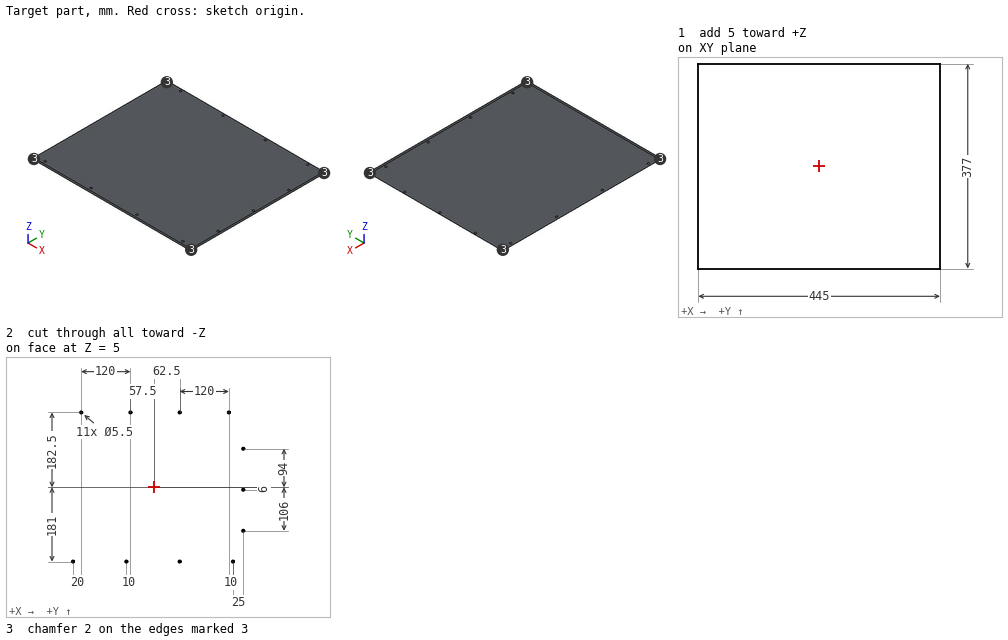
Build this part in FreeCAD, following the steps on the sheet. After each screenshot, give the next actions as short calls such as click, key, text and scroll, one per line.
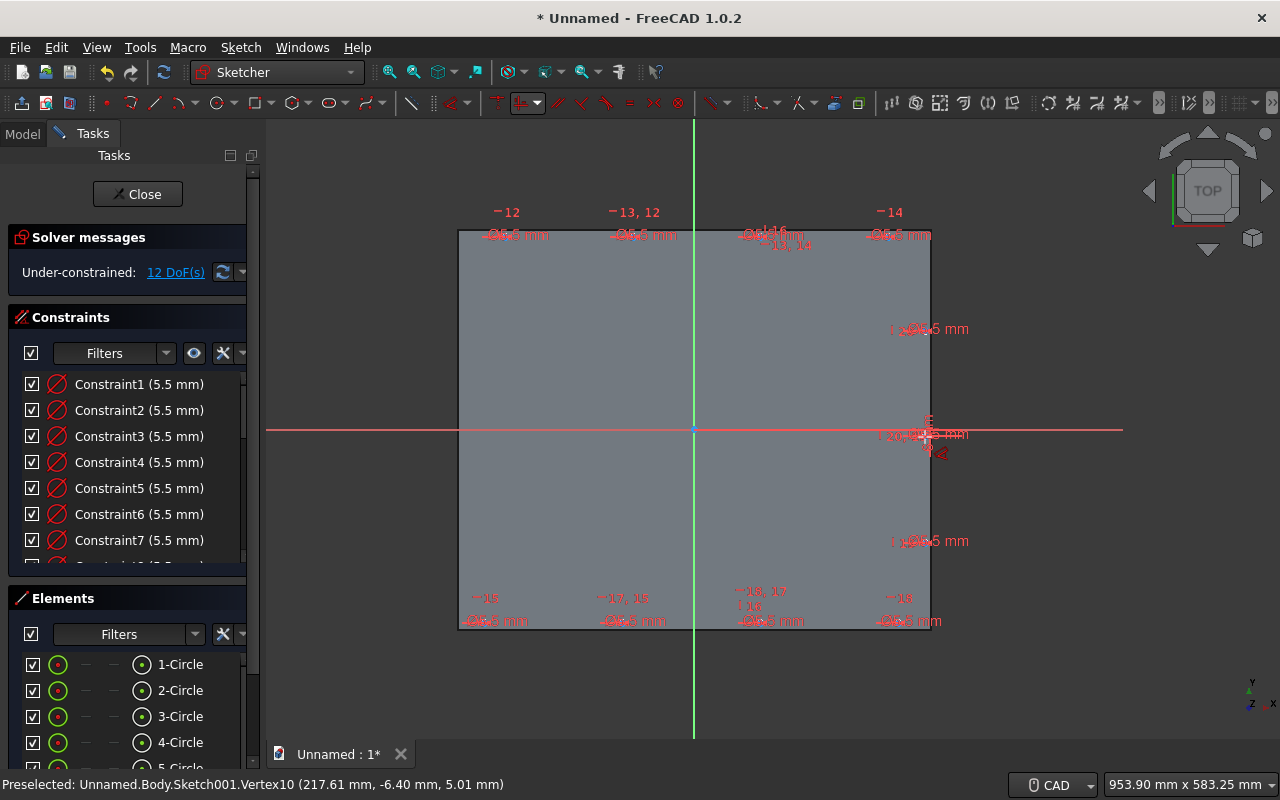
click(925, 331)
click(959, 380)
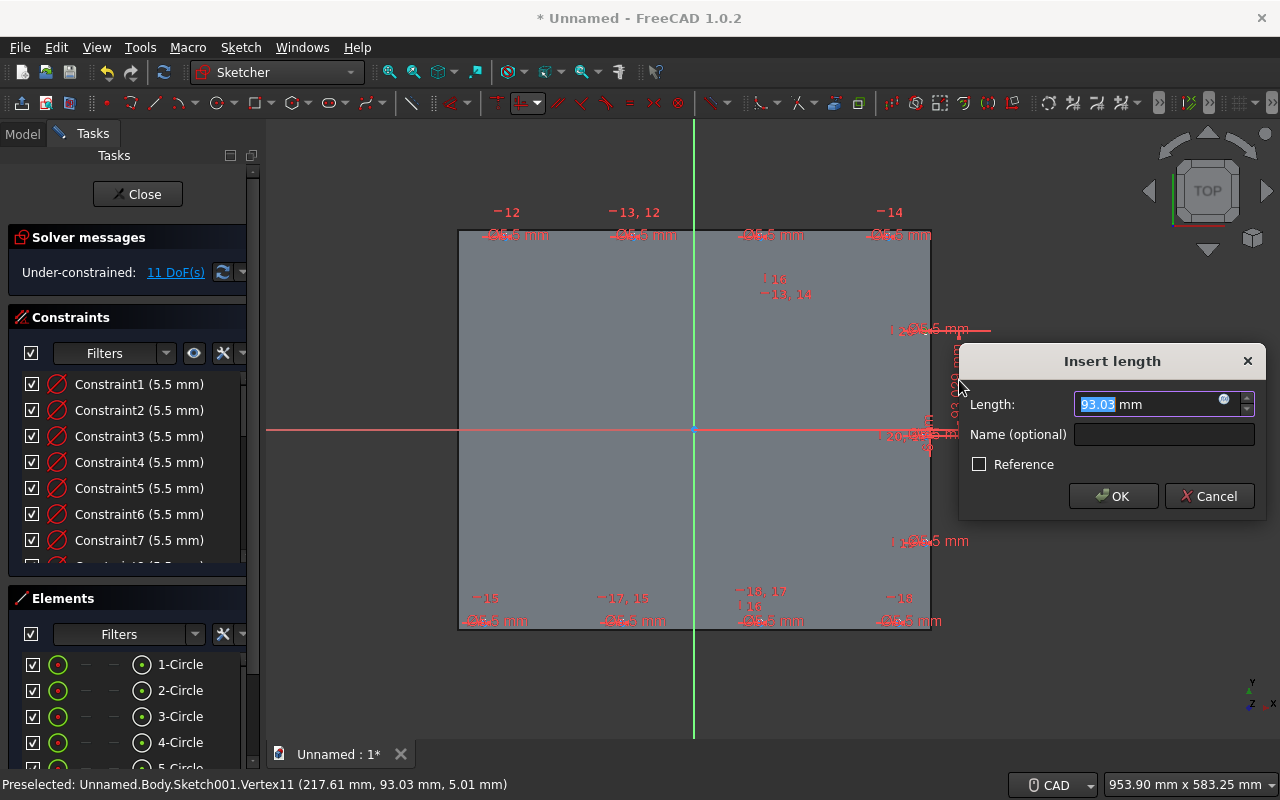
text(94)
key(Return)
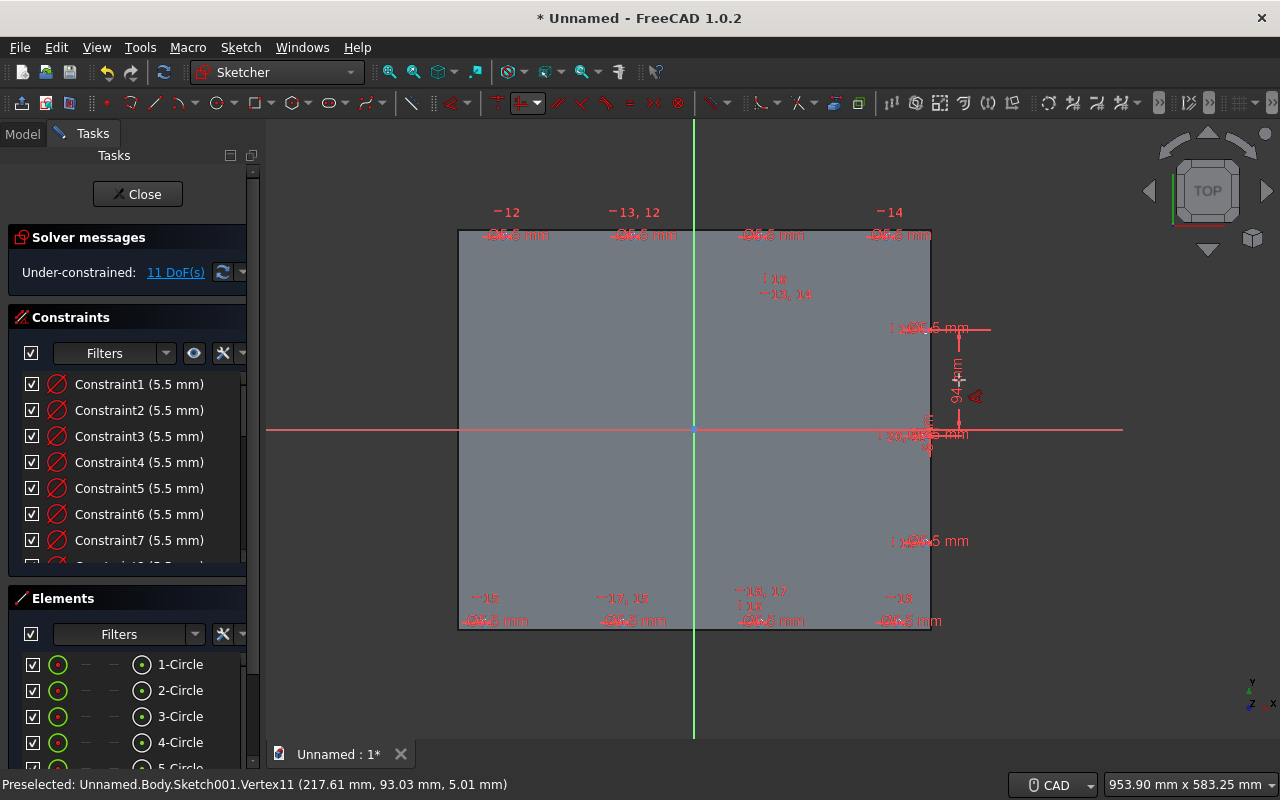
click(484, 623)
click(450, 526)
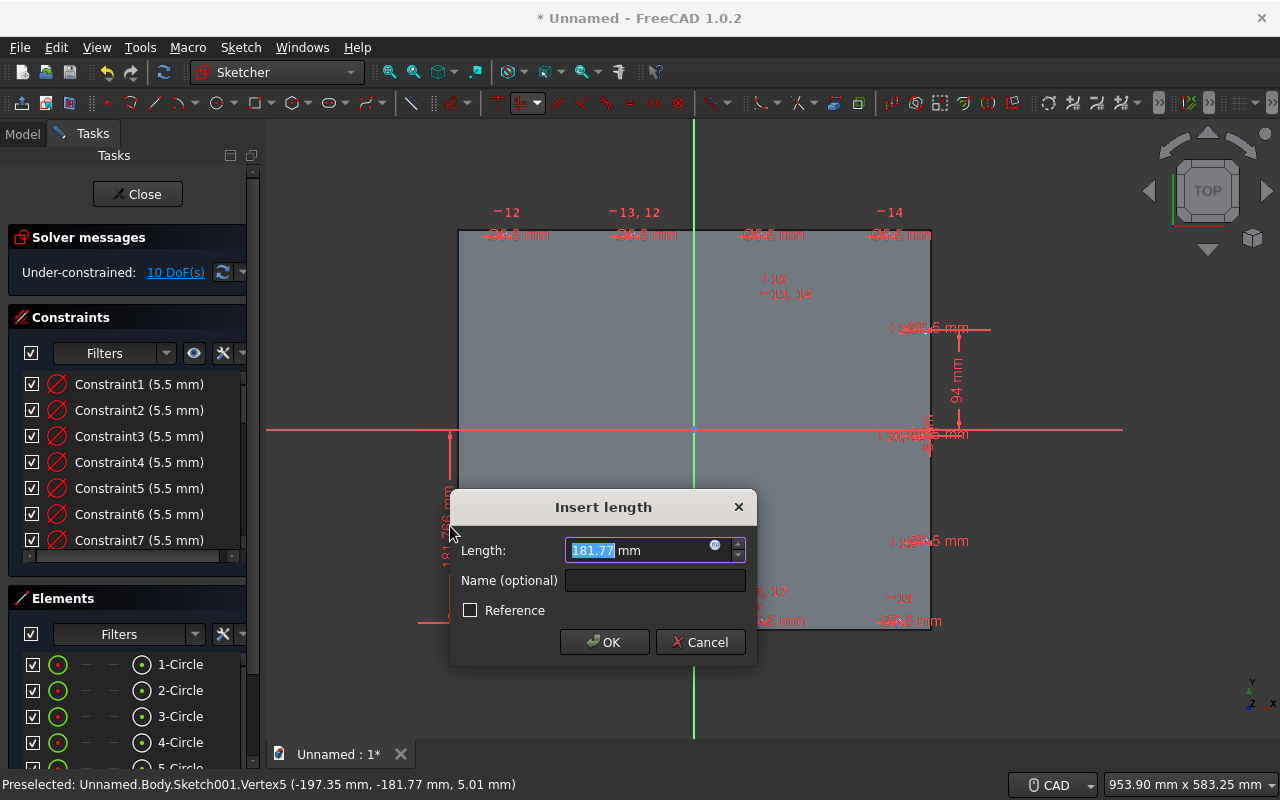
text(181)
key(Return)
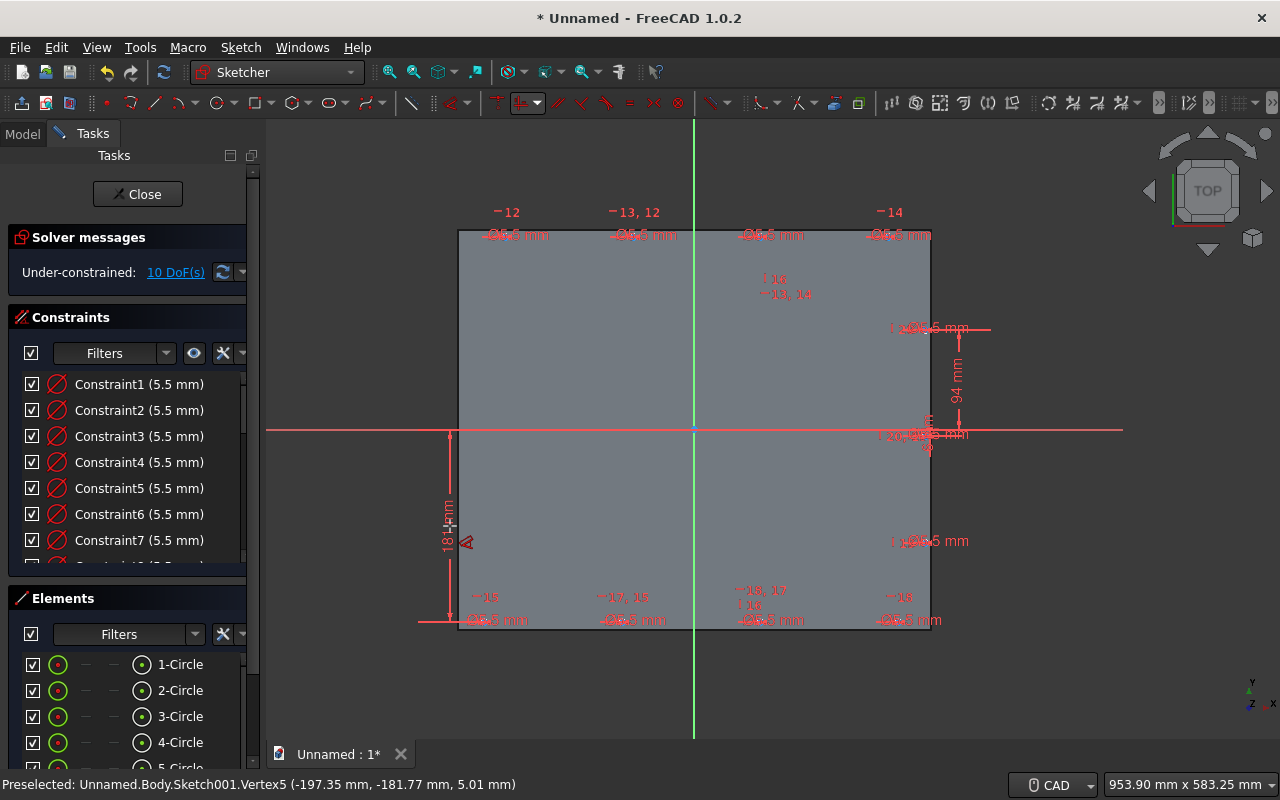
click(925, 543)
click(959, 486)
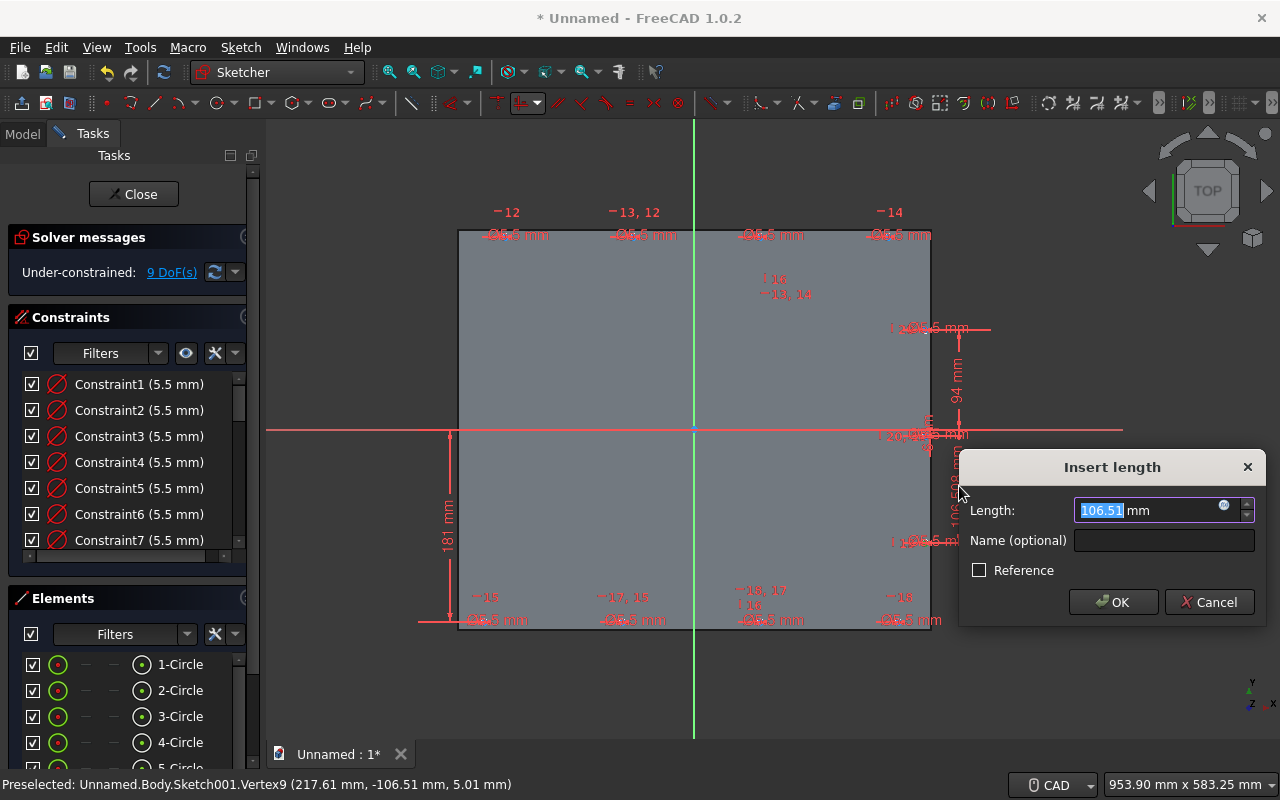
text(106)
key(Return)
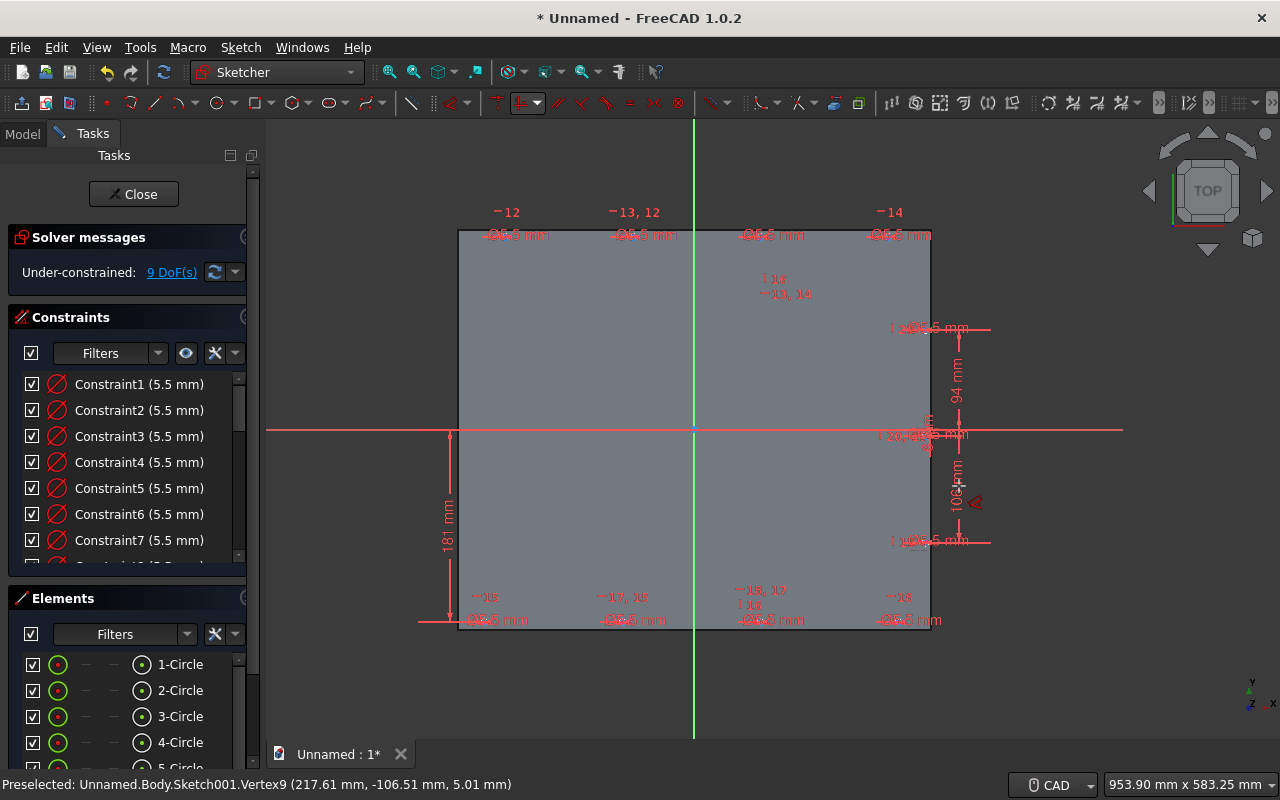
scroll(505, 237, up, 4)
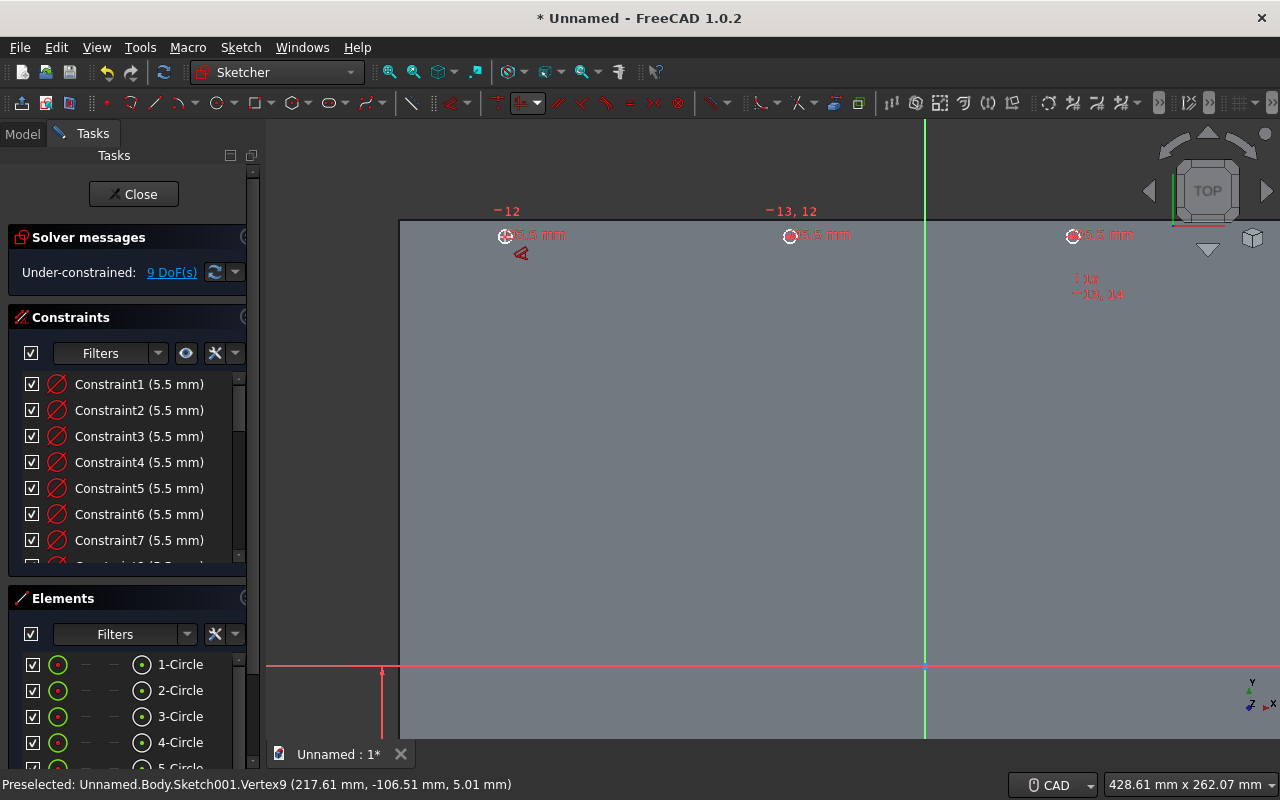
click(505, 237)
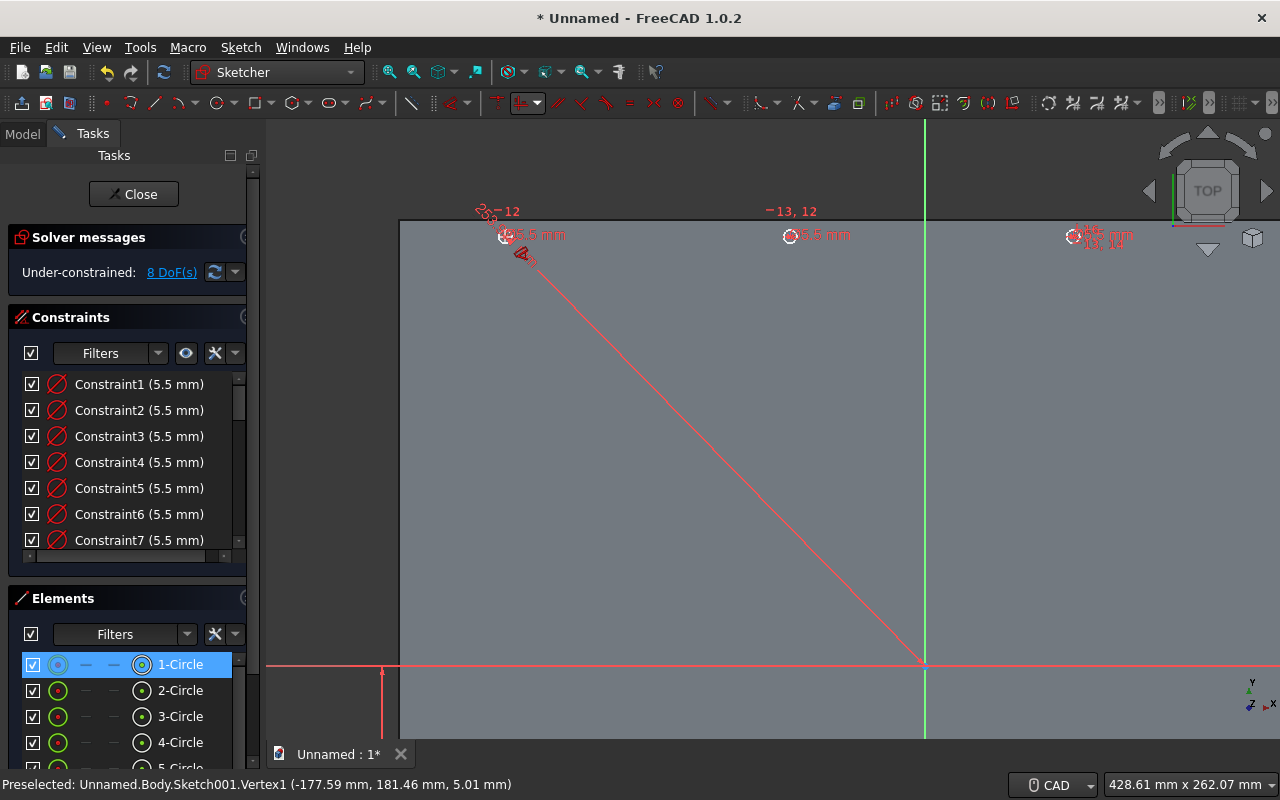
scroll(505, 237, down, 4)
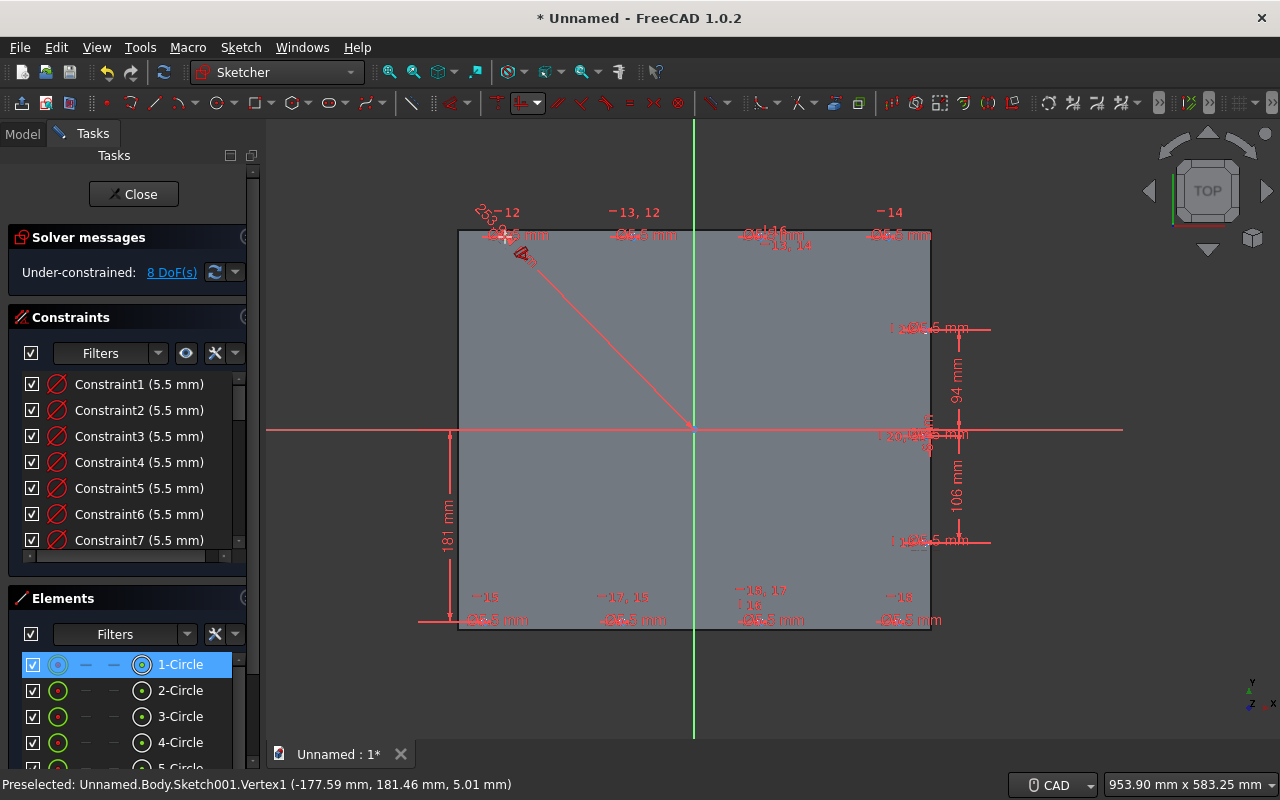
scroll(484, 622, up, 4)